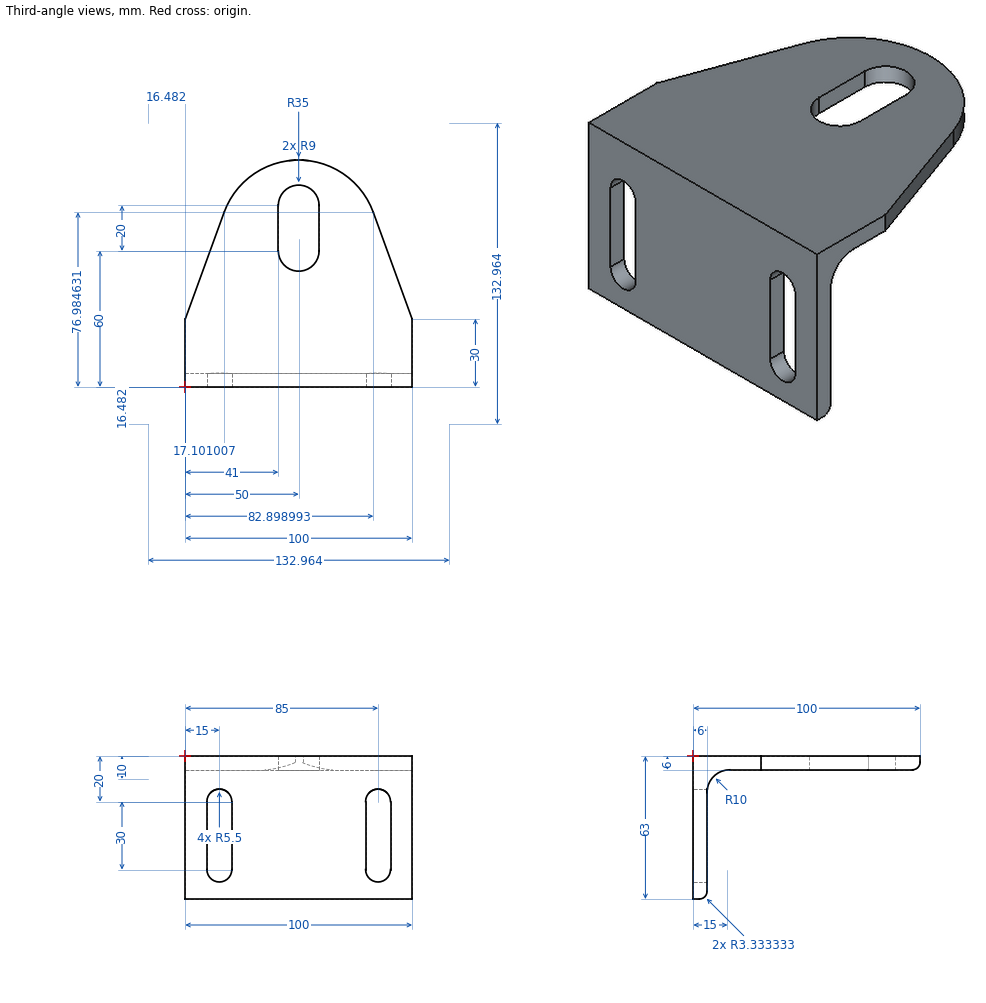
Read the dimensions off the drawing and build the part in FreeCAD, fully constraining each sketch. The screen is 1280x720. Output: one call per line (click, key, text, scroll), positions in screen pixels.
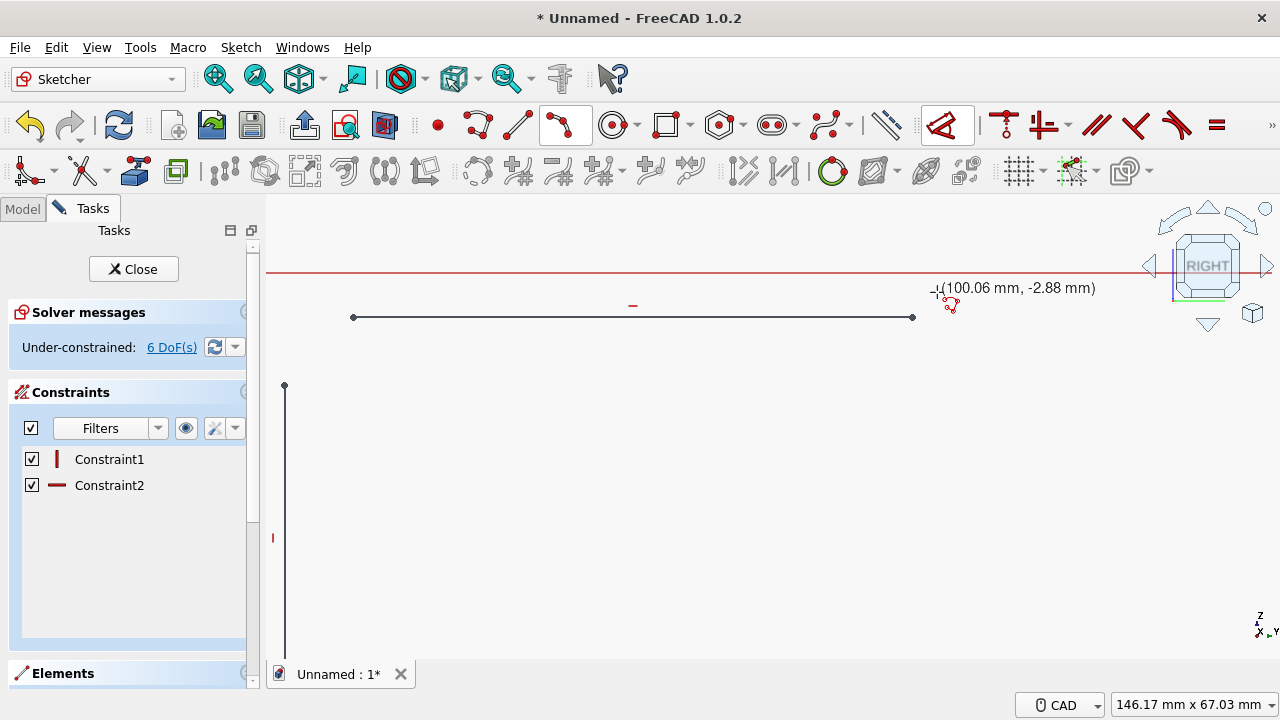
click(936, 292)
click(936, 273)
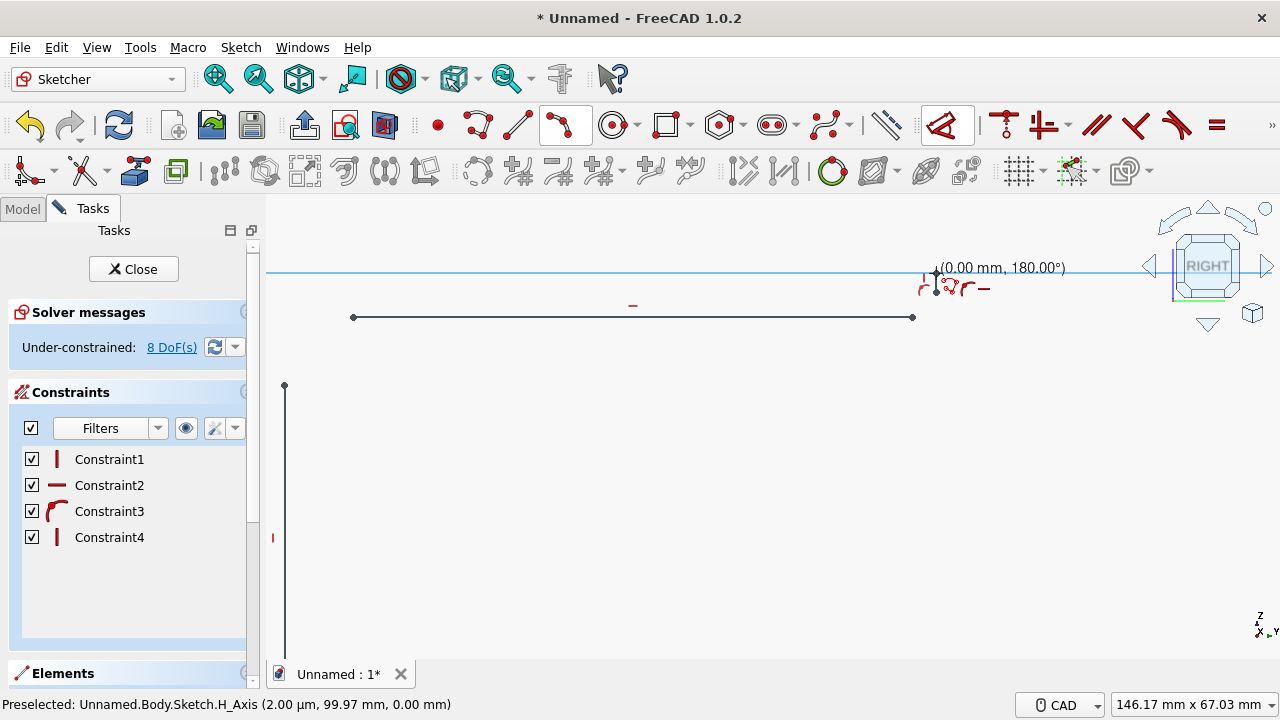
scroll(939, 293, down, 2)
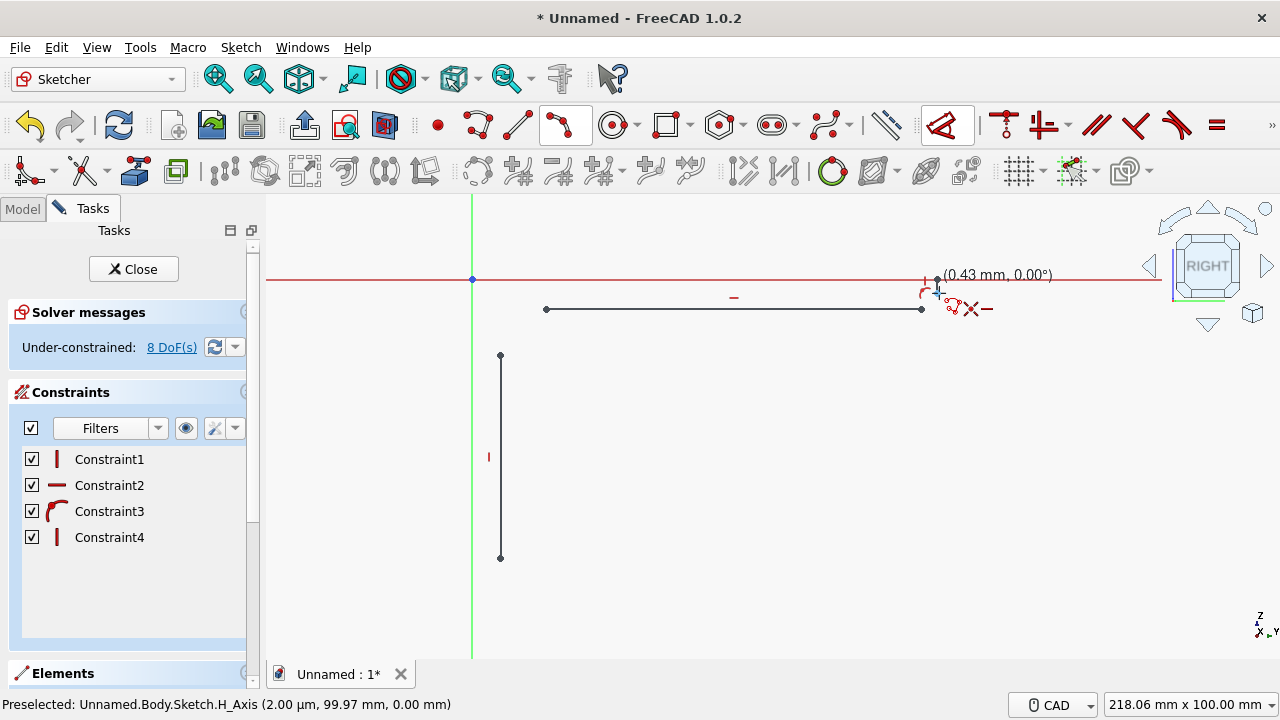
click(472, 280)
click(481, 573)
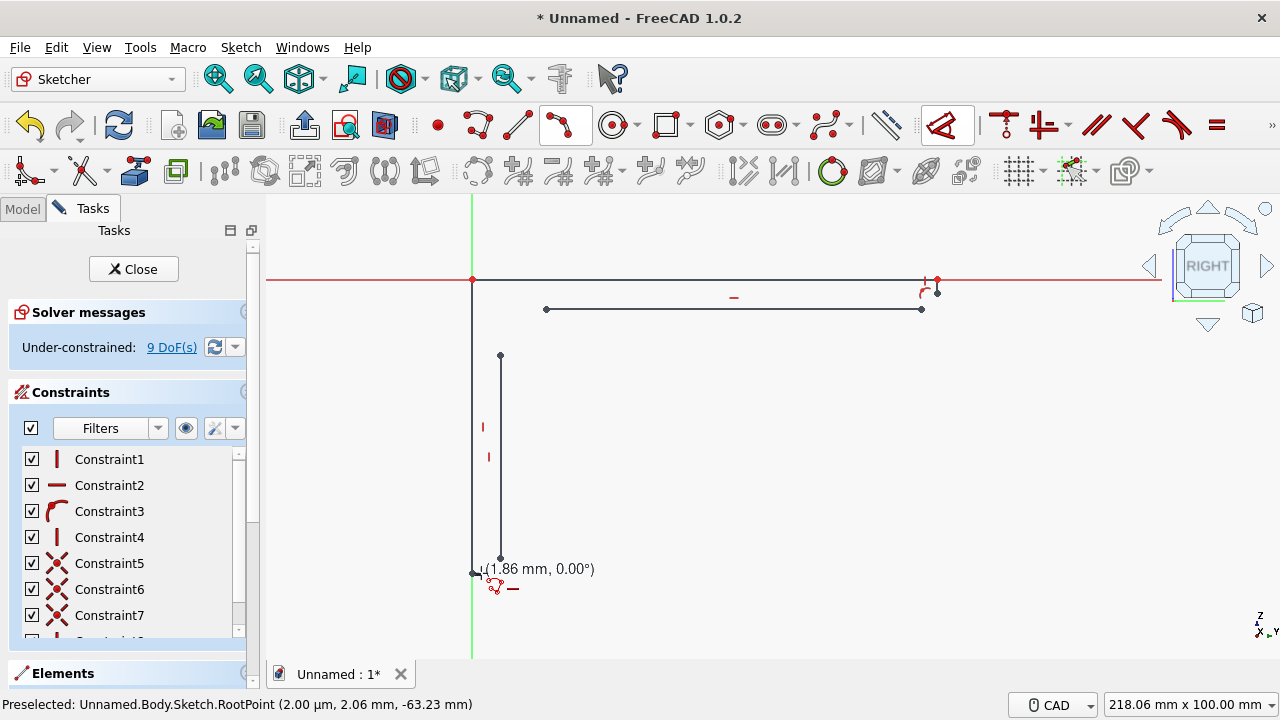
scroll(485, 573, up, 2)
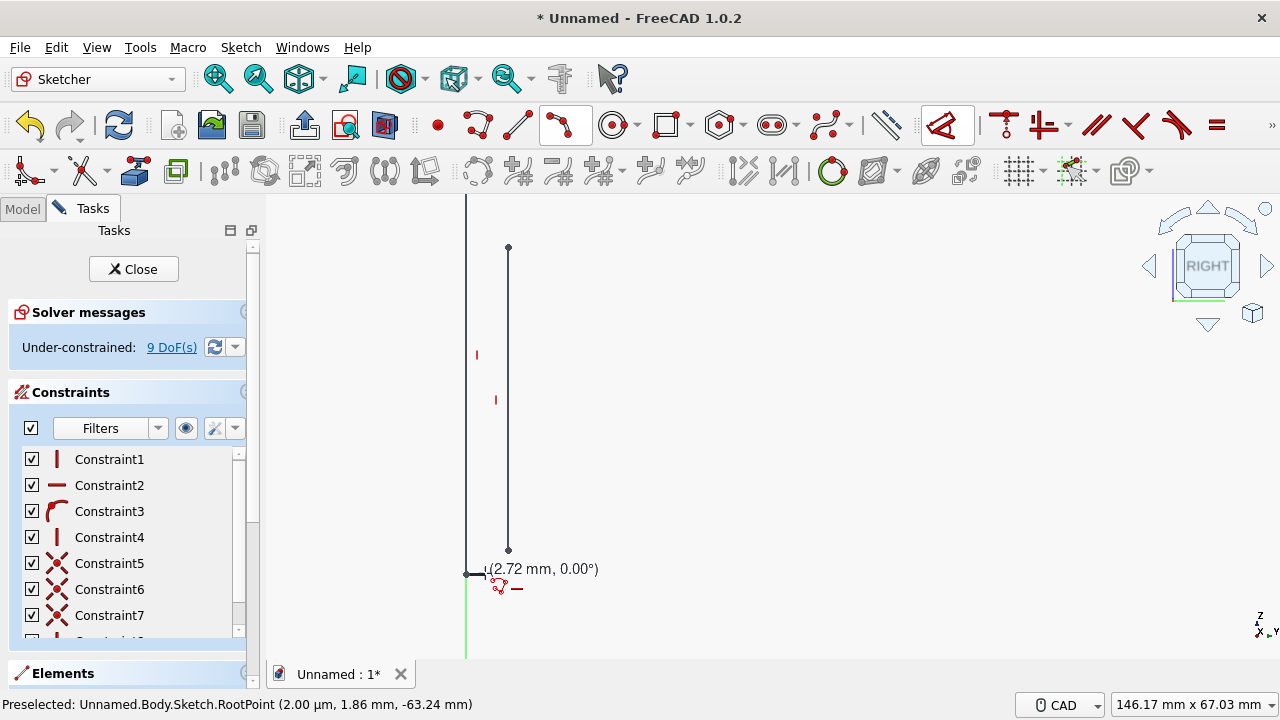
click(485, 573)
right_click(485, 573)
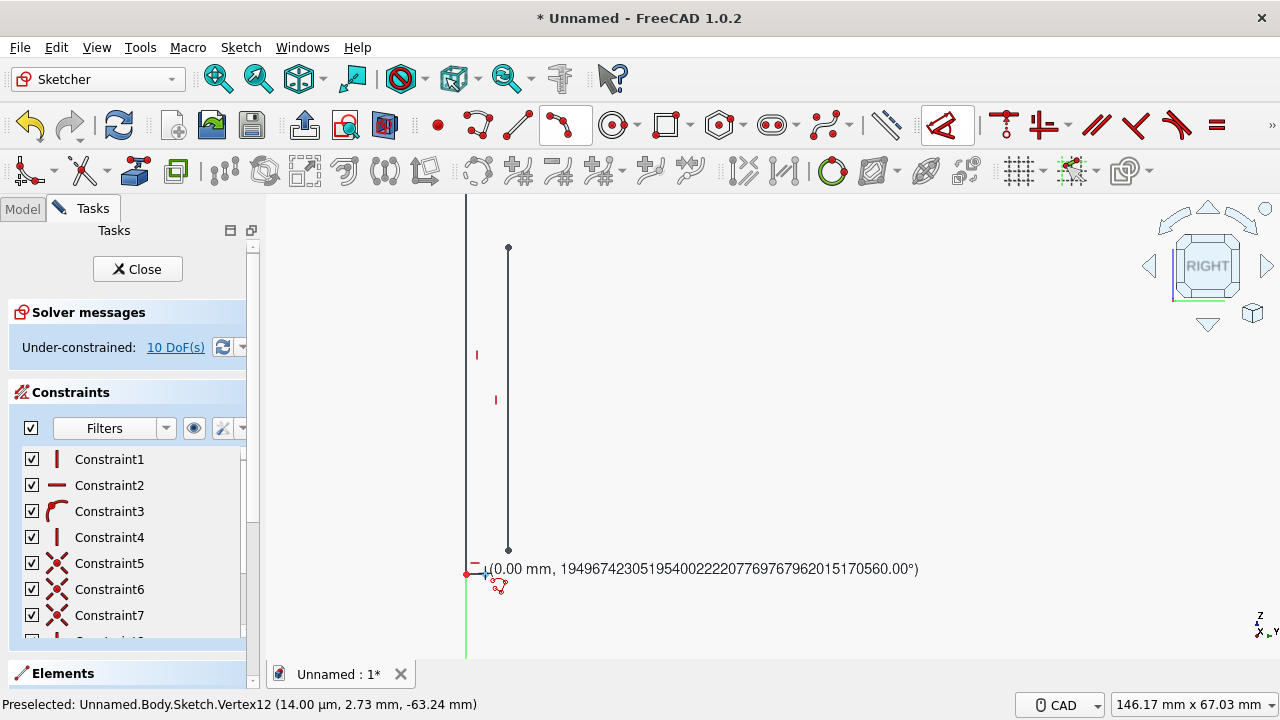
click(560, 126)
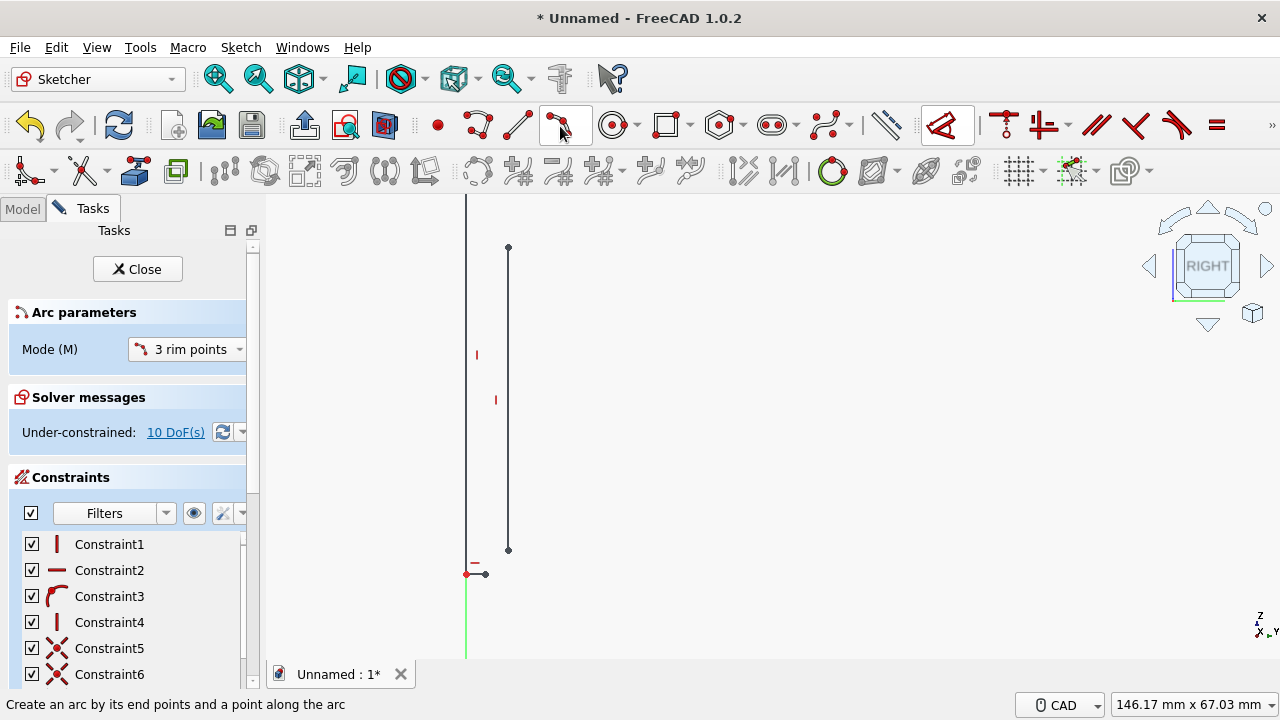
click(508, 248)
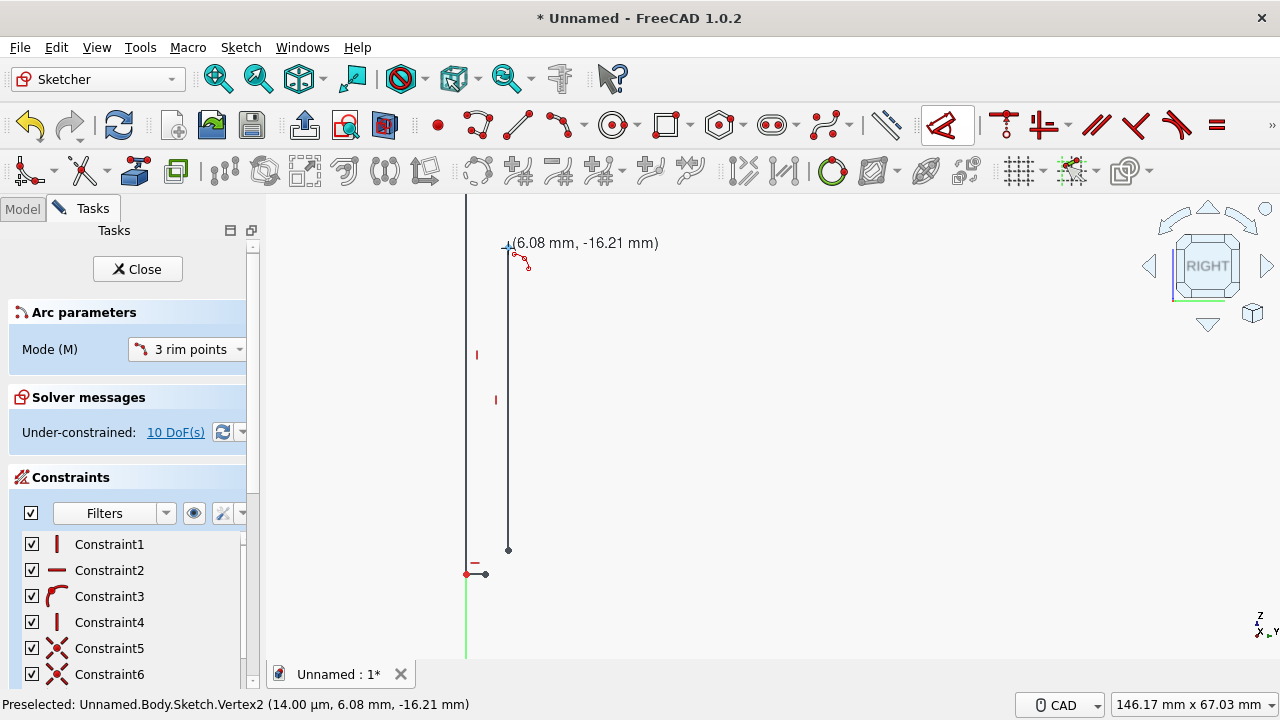
scroll(484, 574, down, 2)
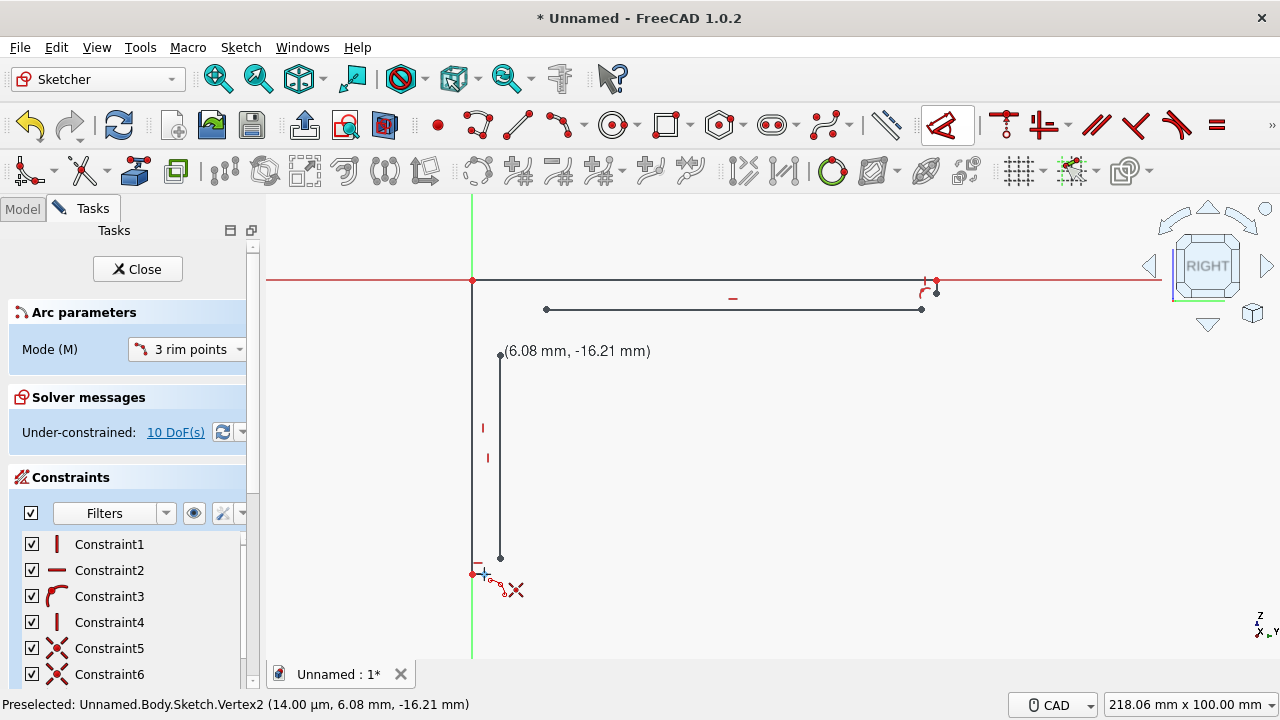
click(546, 310)
click(514, 322)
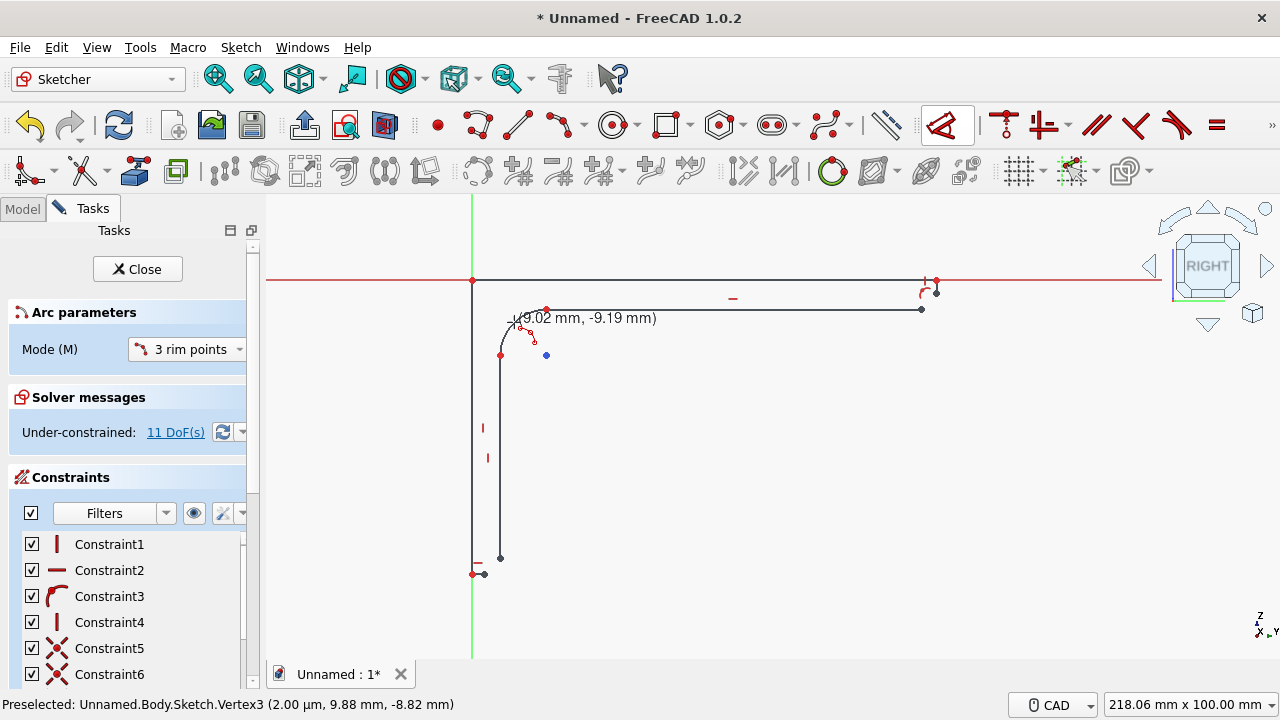
click(921, 310)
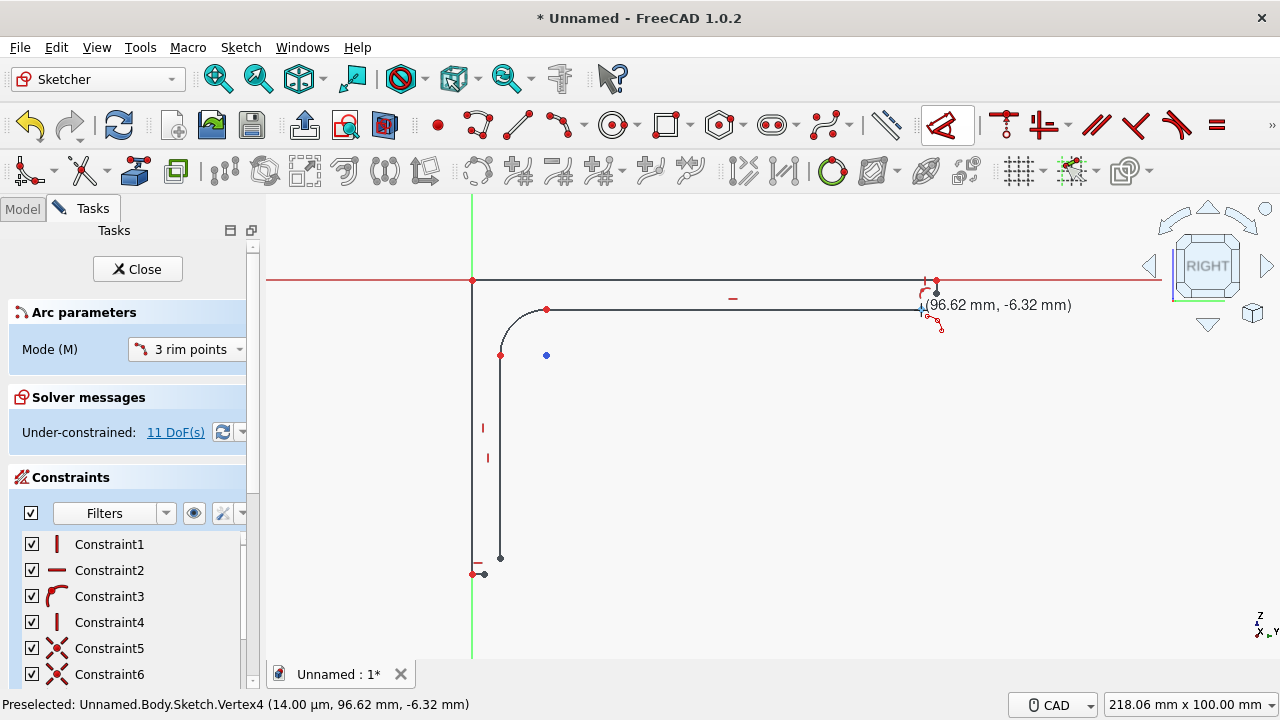
scroll(937, 293, up, 5)